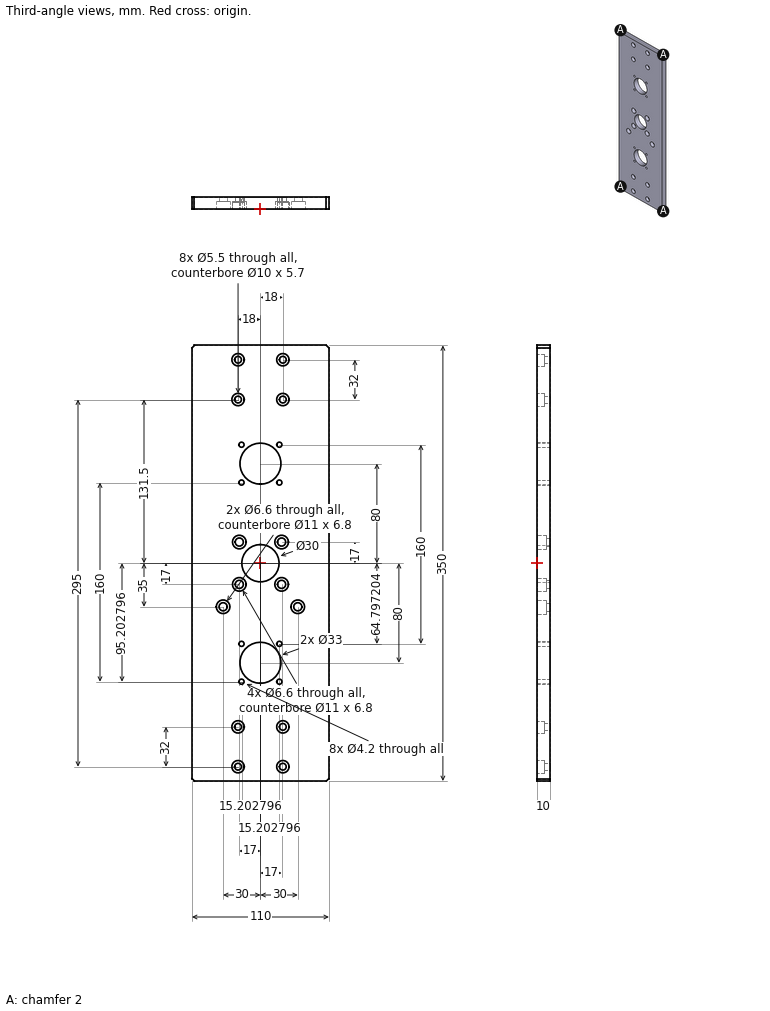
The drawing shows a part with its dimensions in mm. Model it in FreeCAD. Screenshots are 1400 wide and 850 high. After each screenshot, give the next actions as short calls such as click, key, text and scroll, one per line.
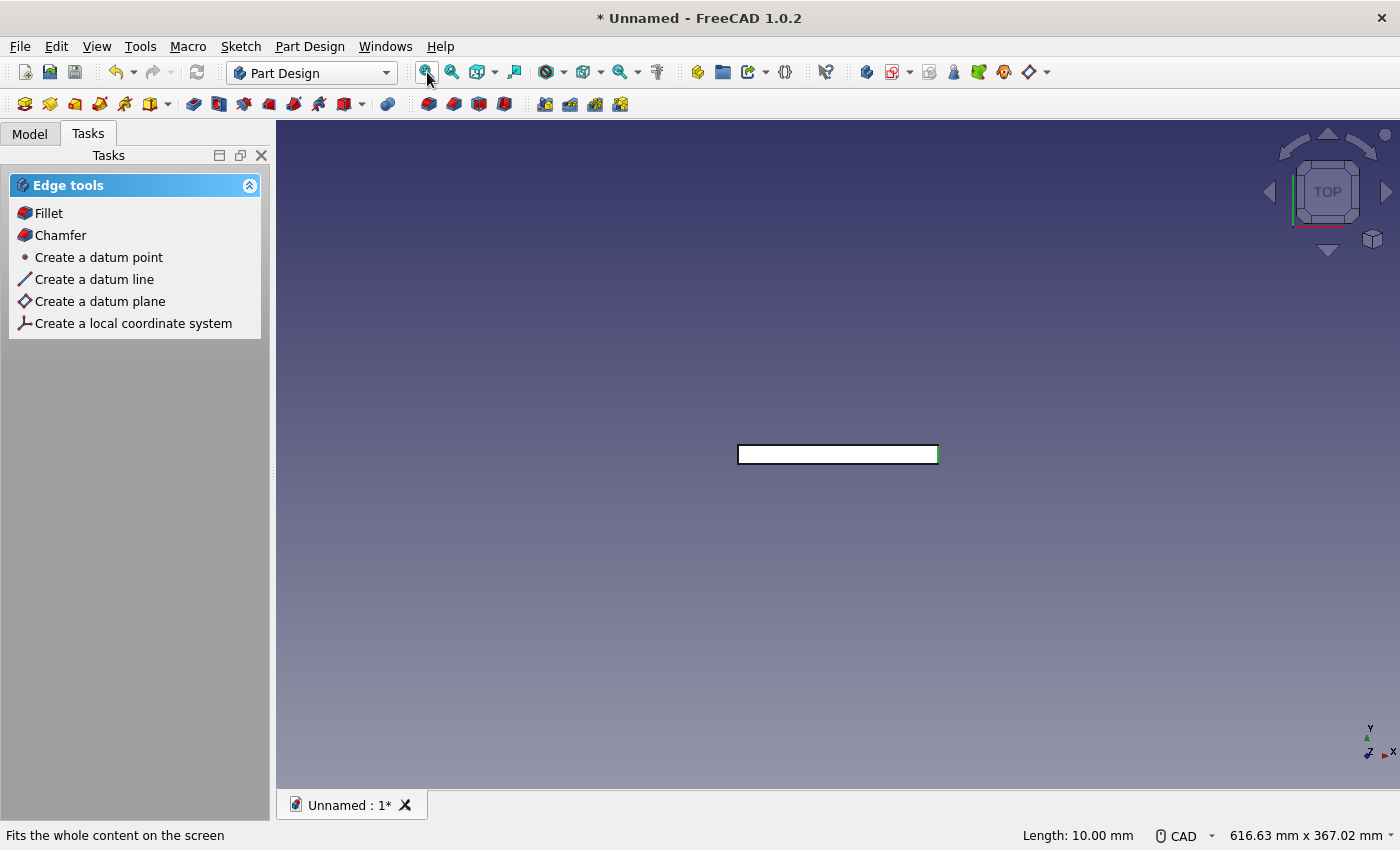
key(v)
key(f)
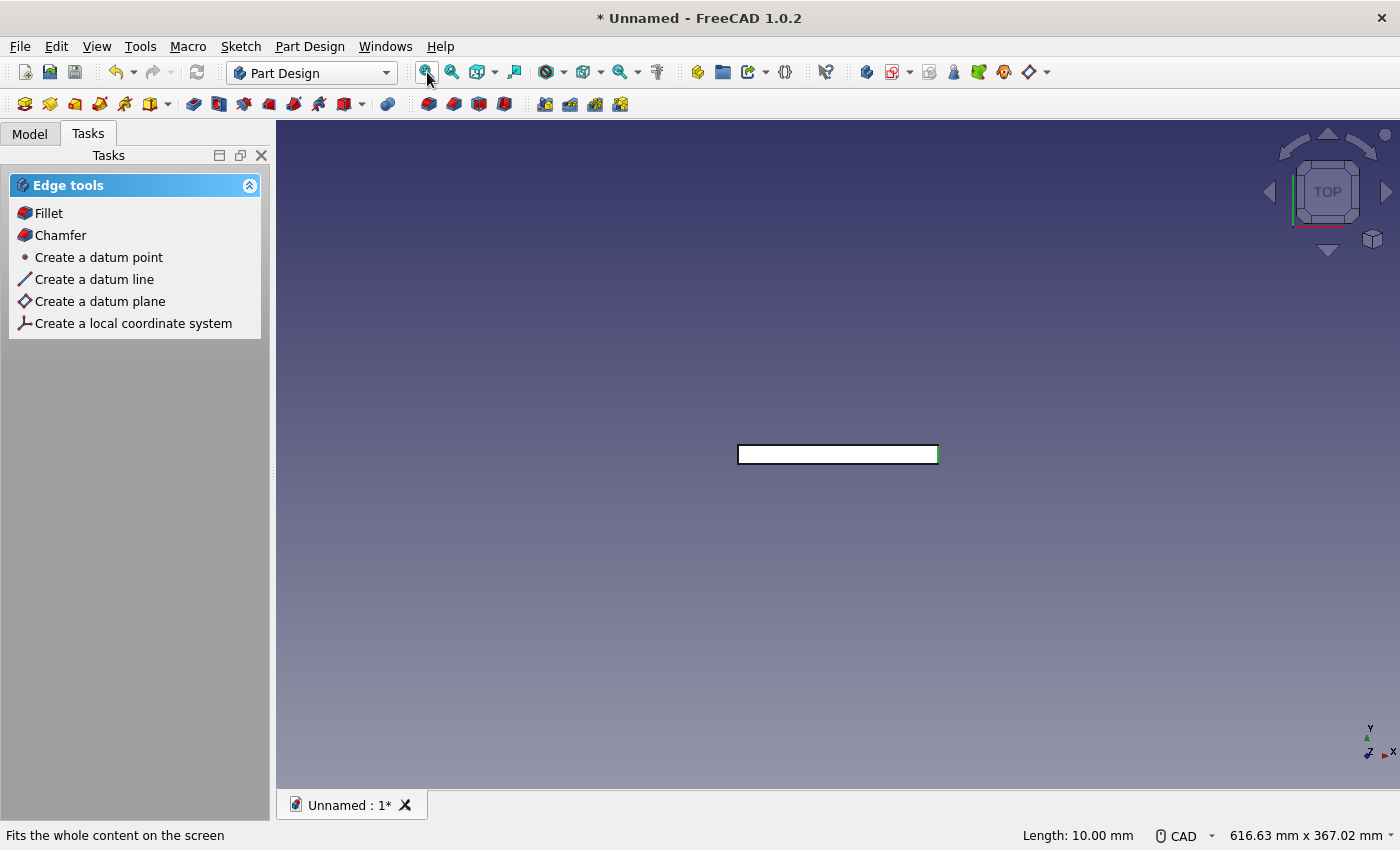
click(738, 453, ctrl)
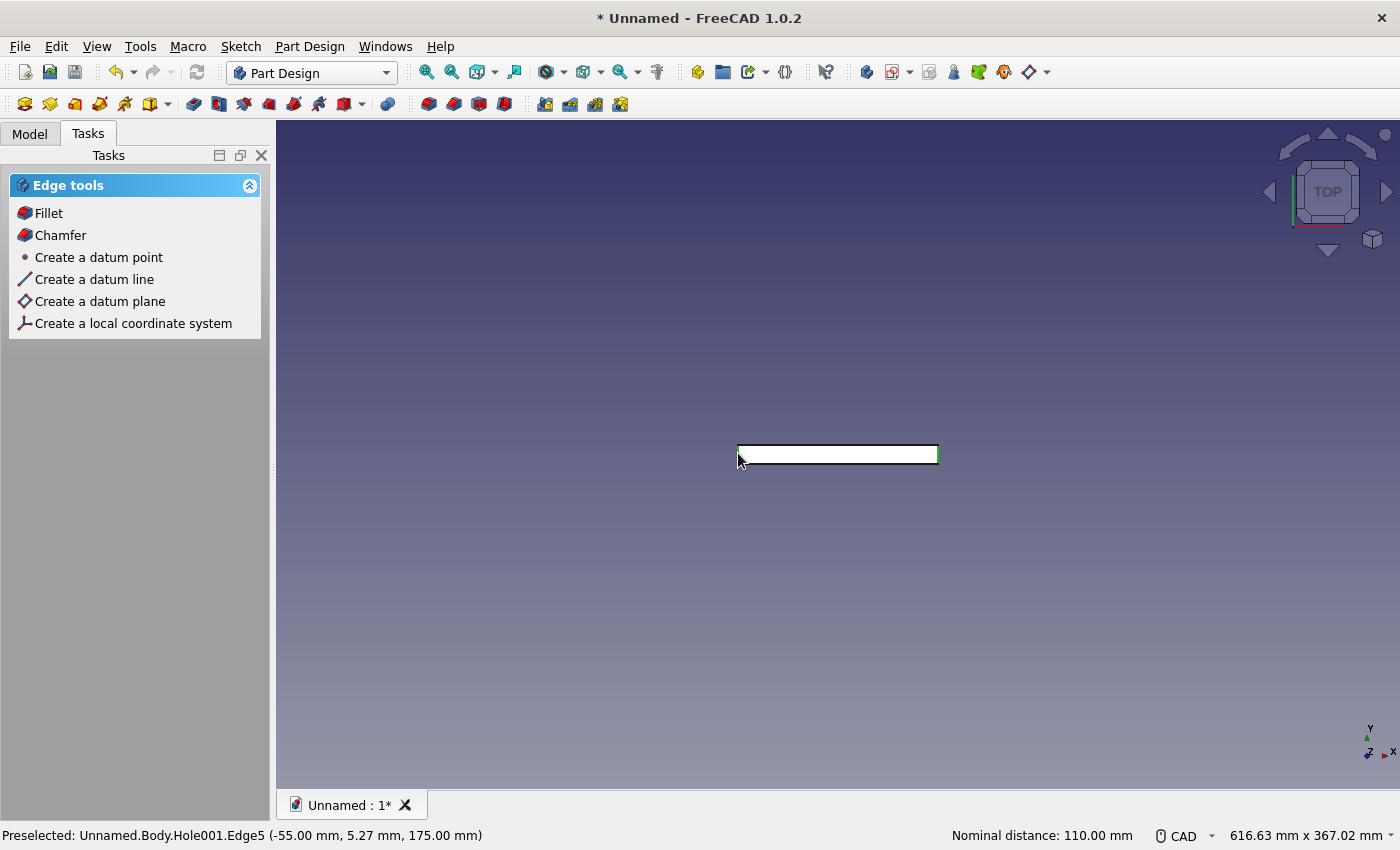
scroll(738, 453, up, 4)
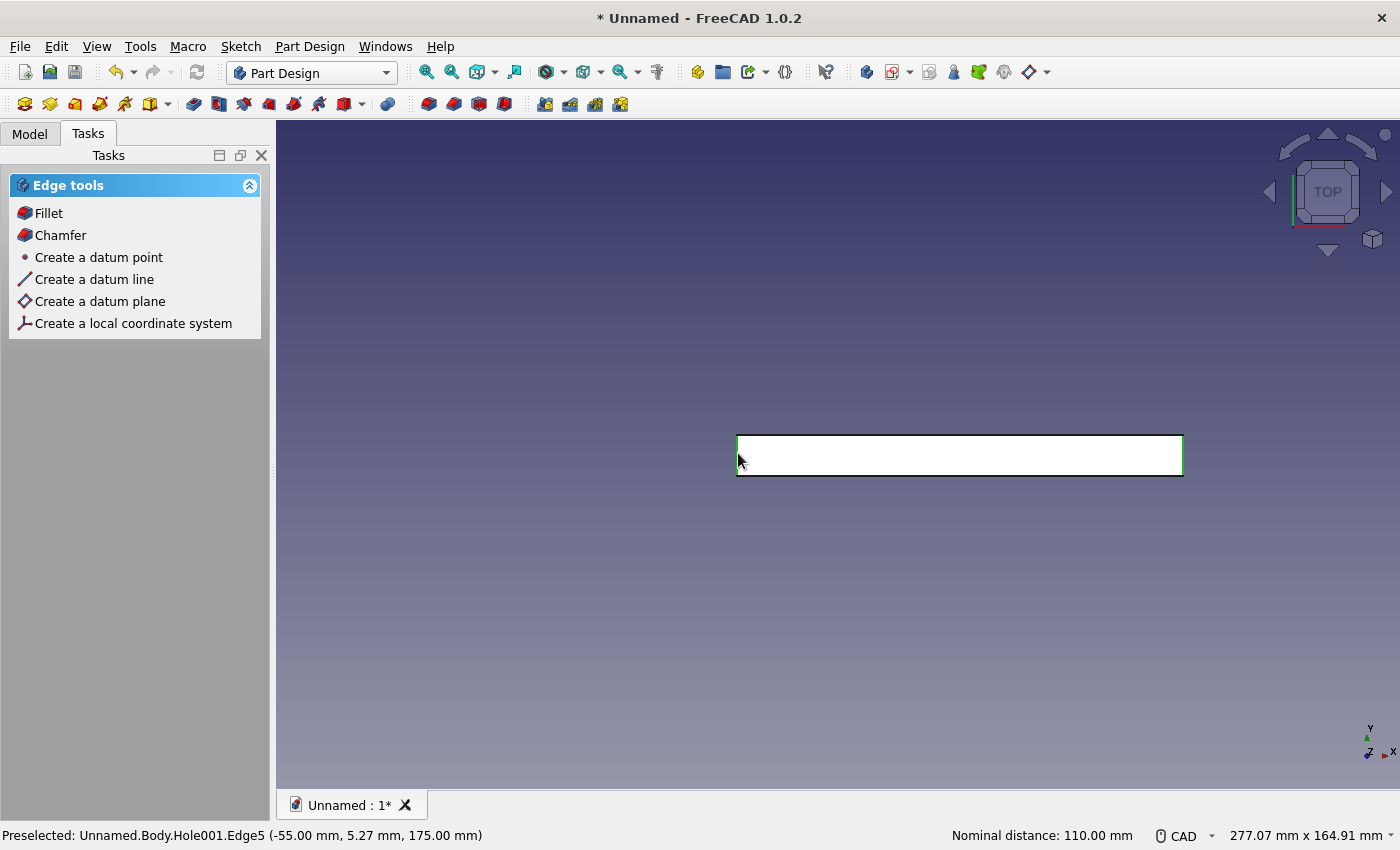
key(v)
key(f)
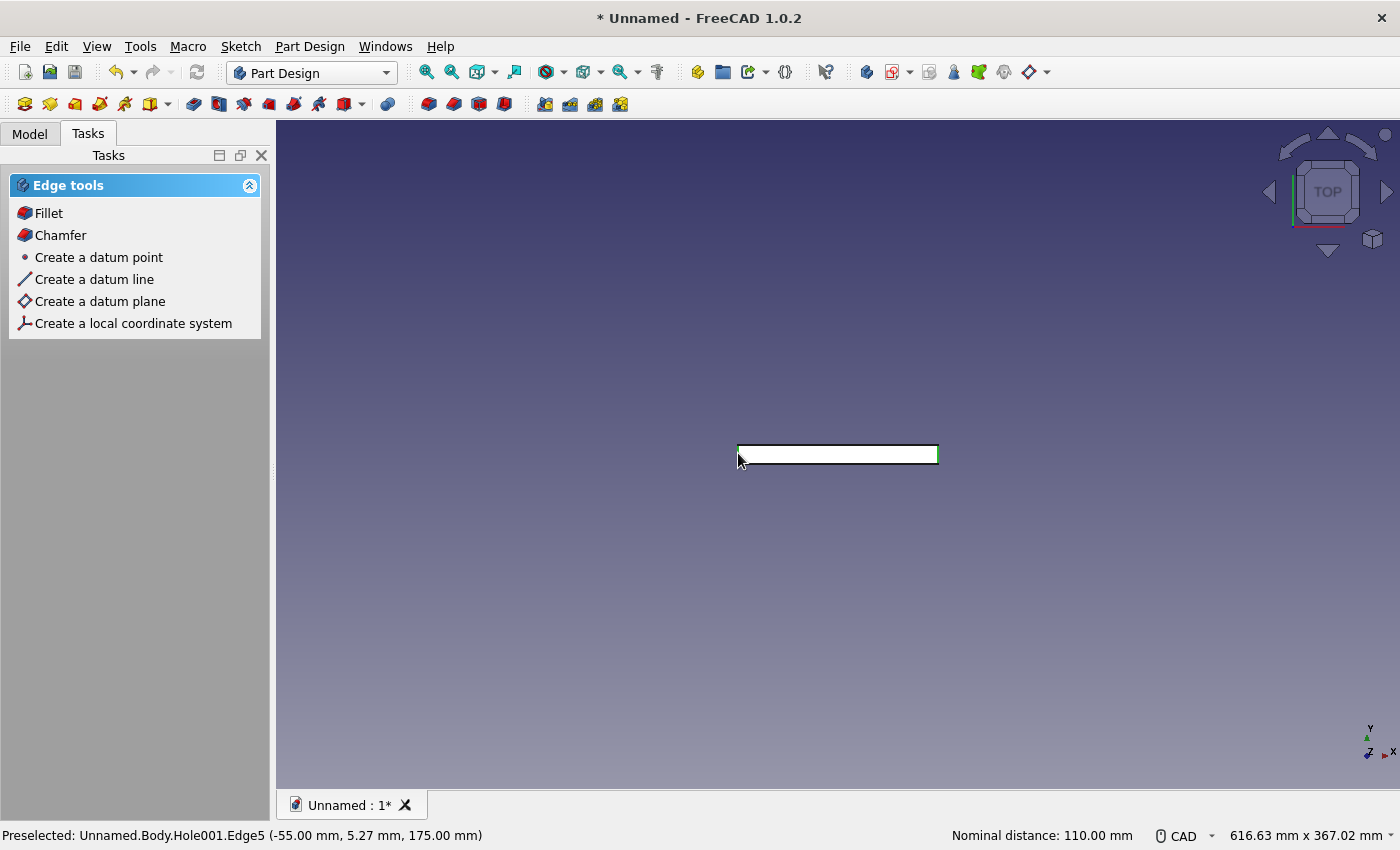
key(1)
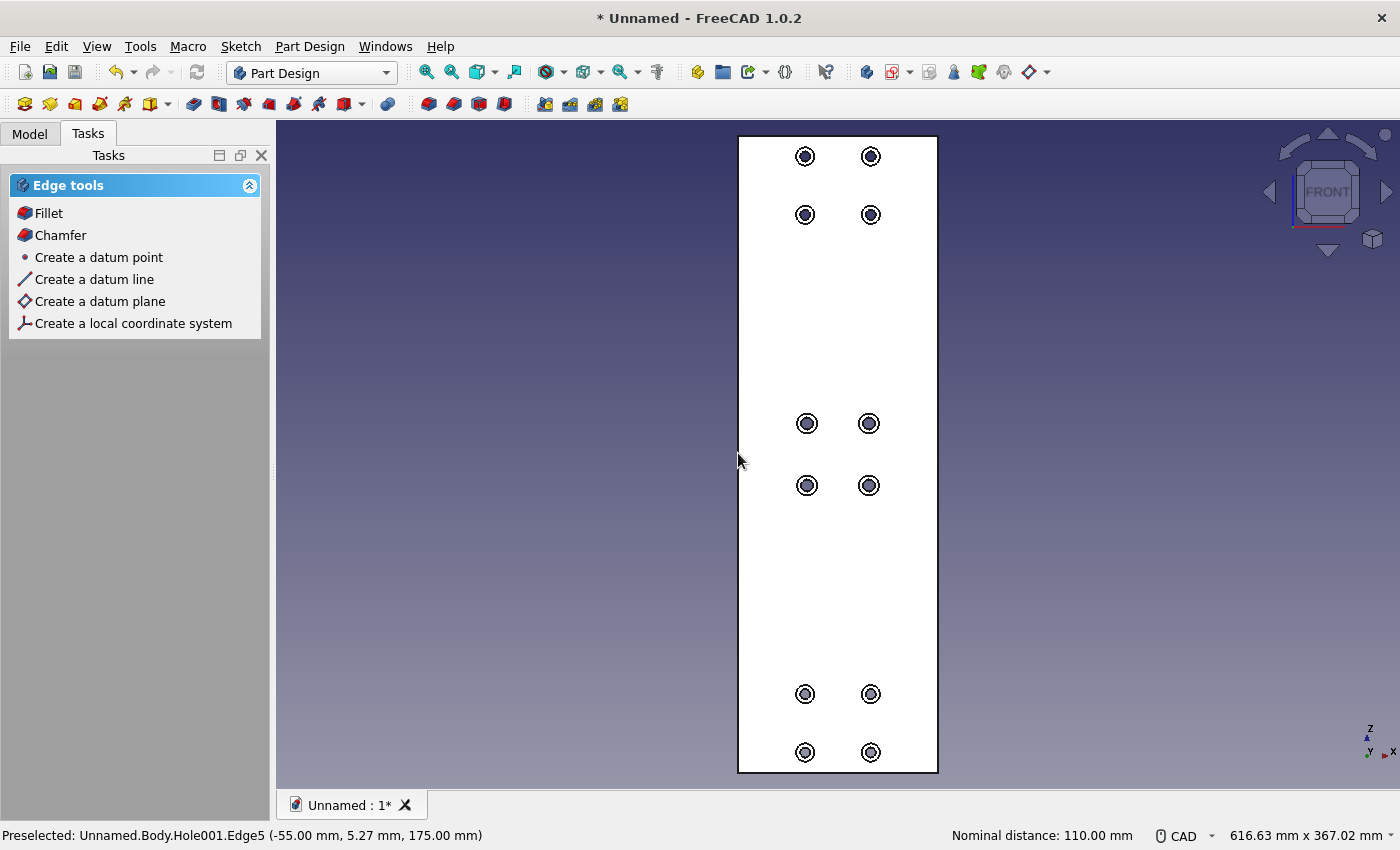
key(3)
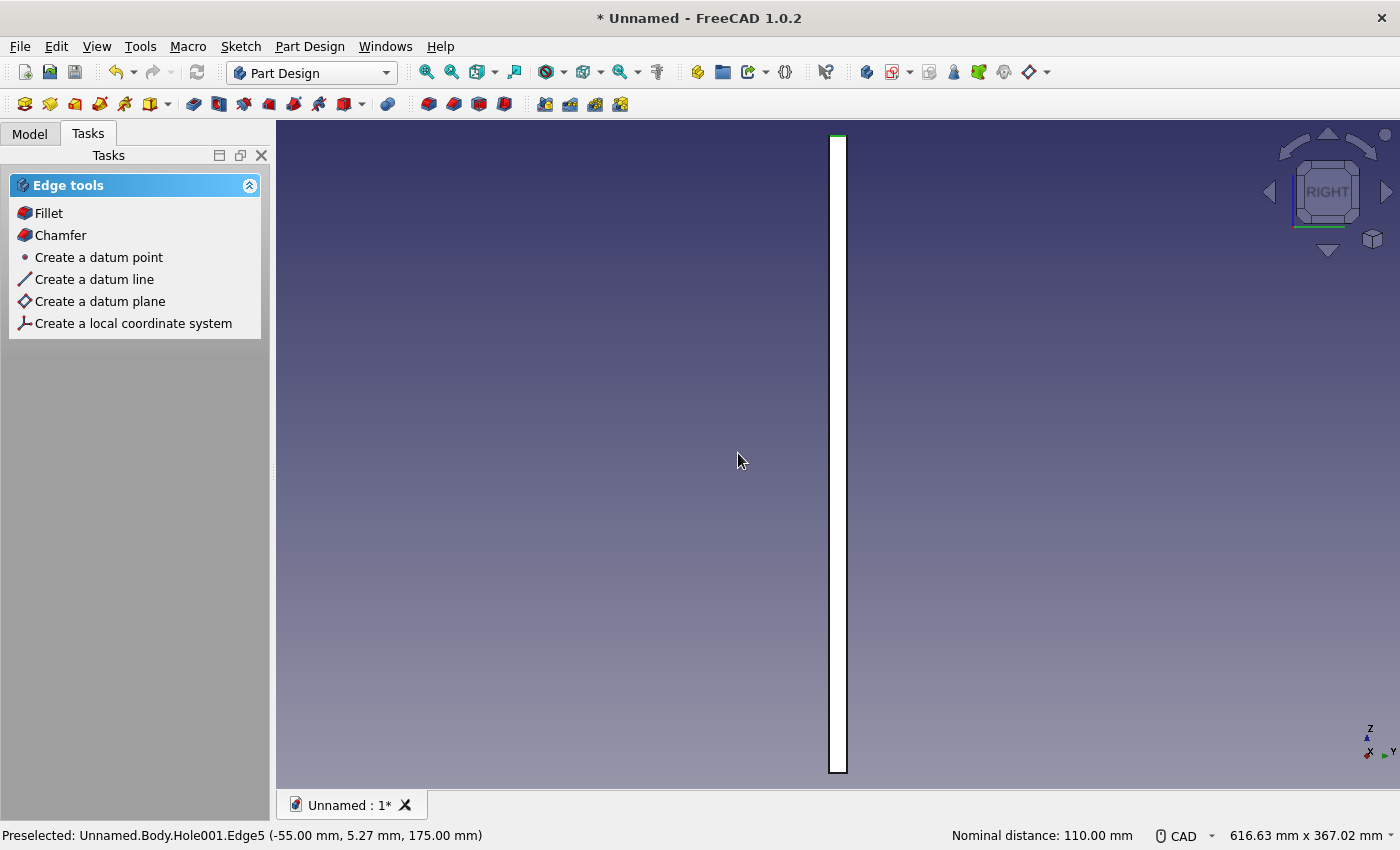
key(5)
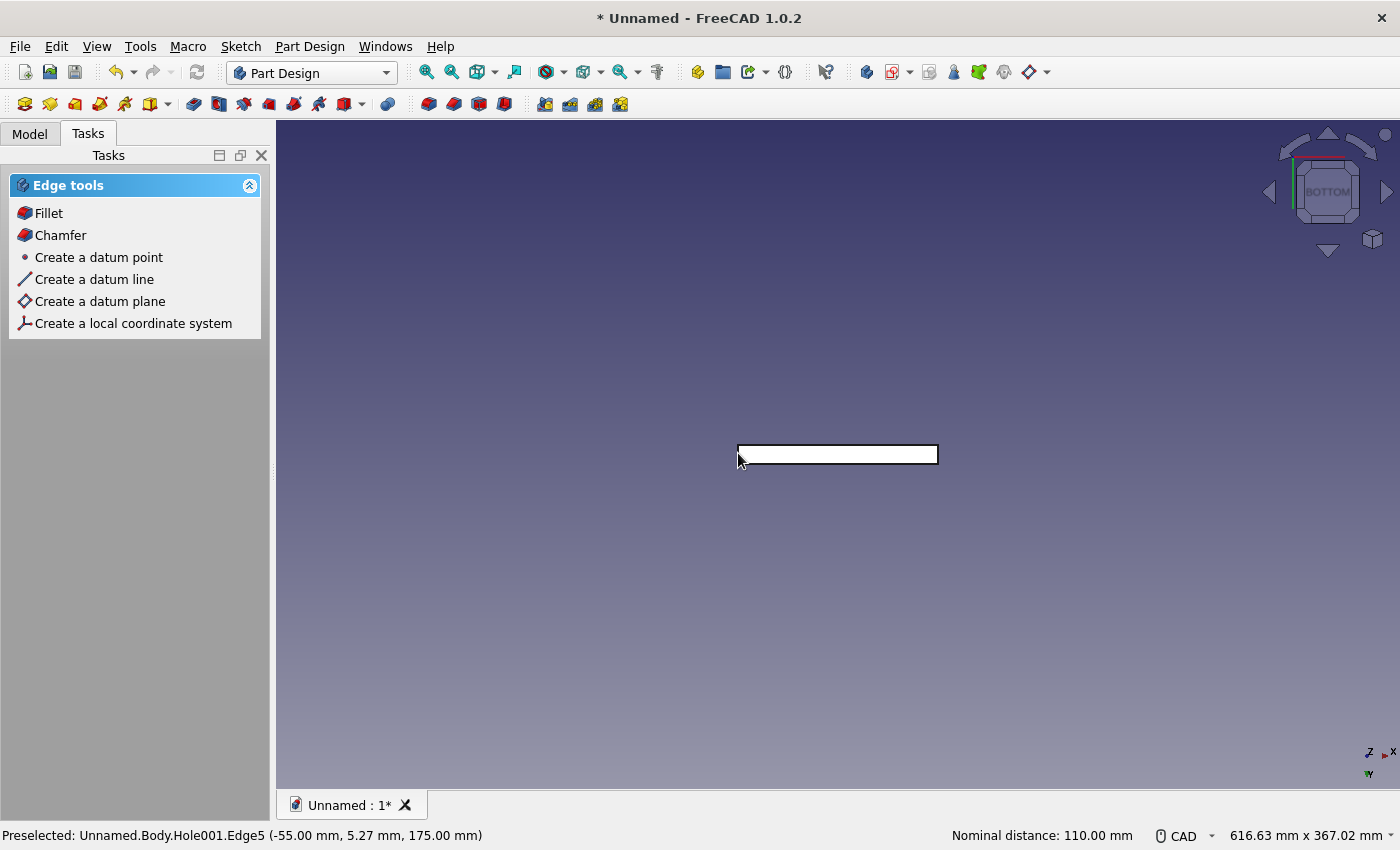
key(v)
key(f)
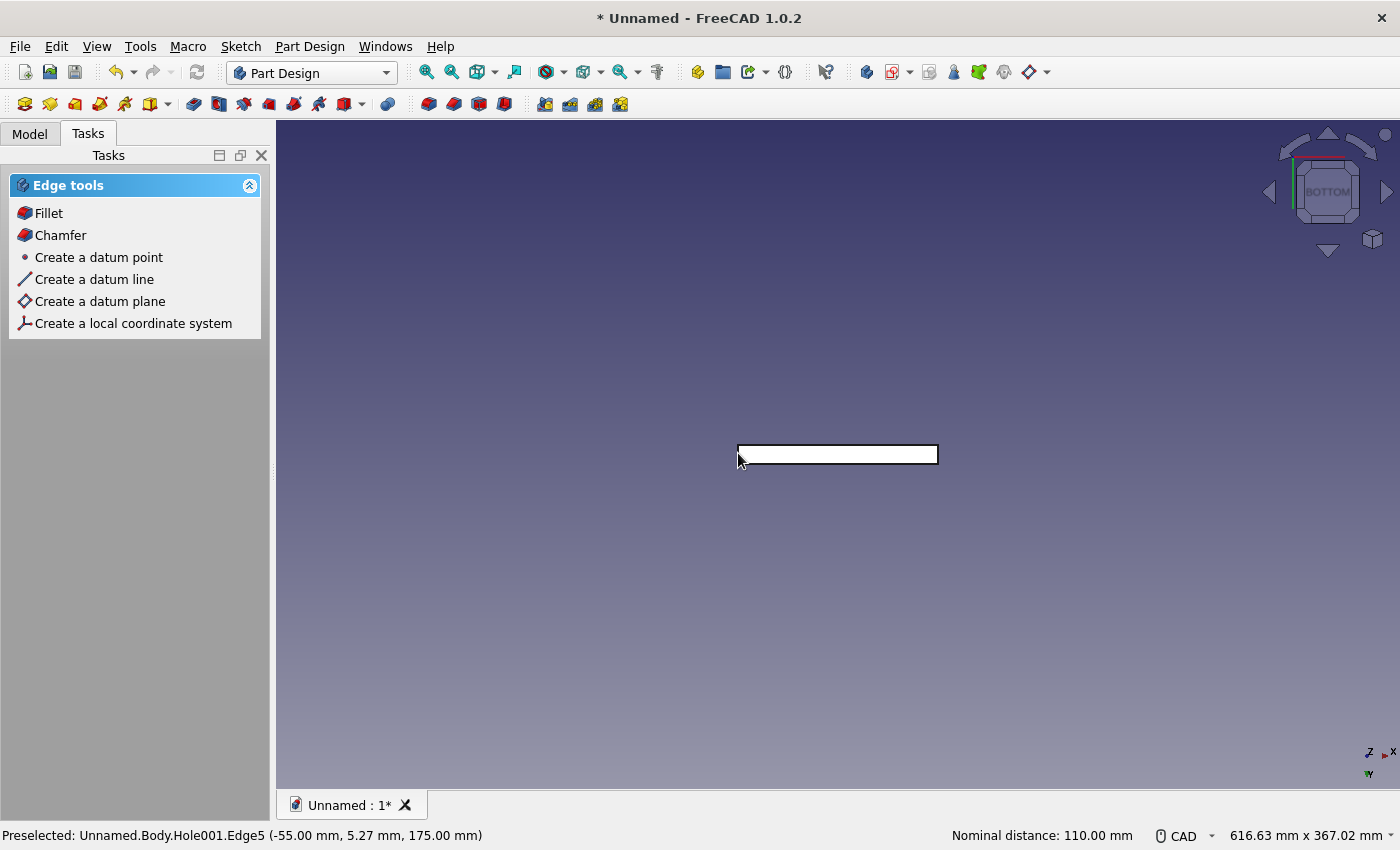
click(738, 453, ctrl)